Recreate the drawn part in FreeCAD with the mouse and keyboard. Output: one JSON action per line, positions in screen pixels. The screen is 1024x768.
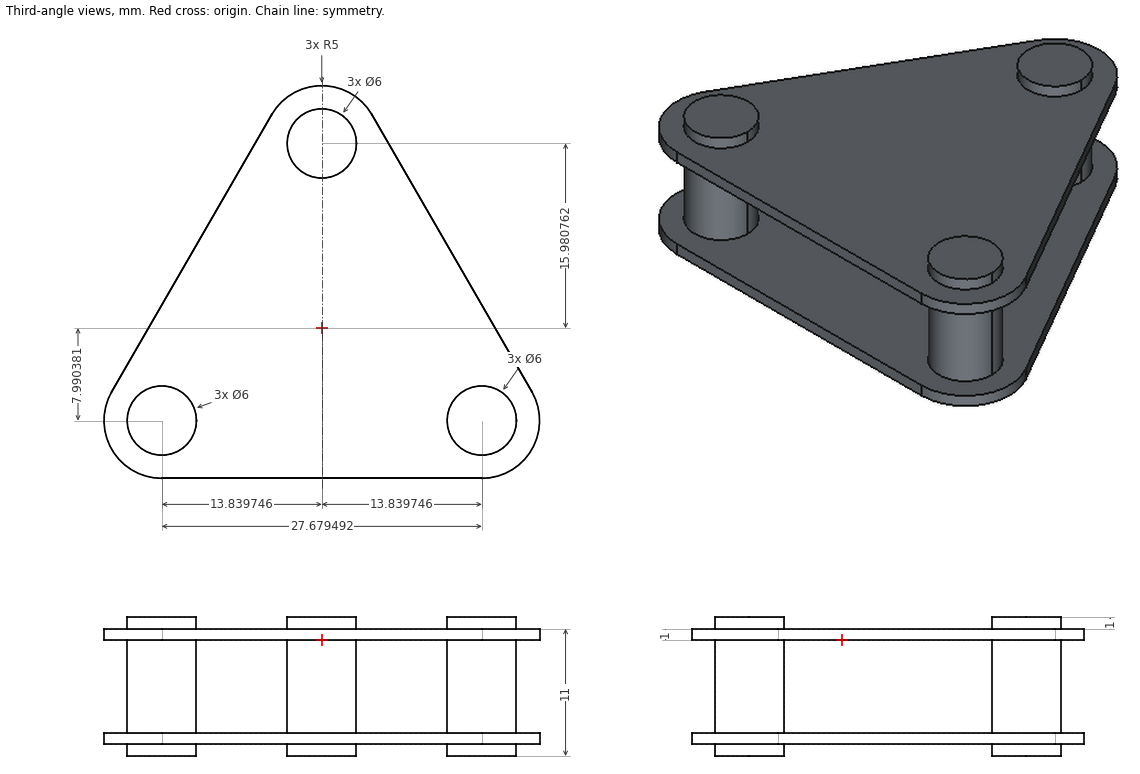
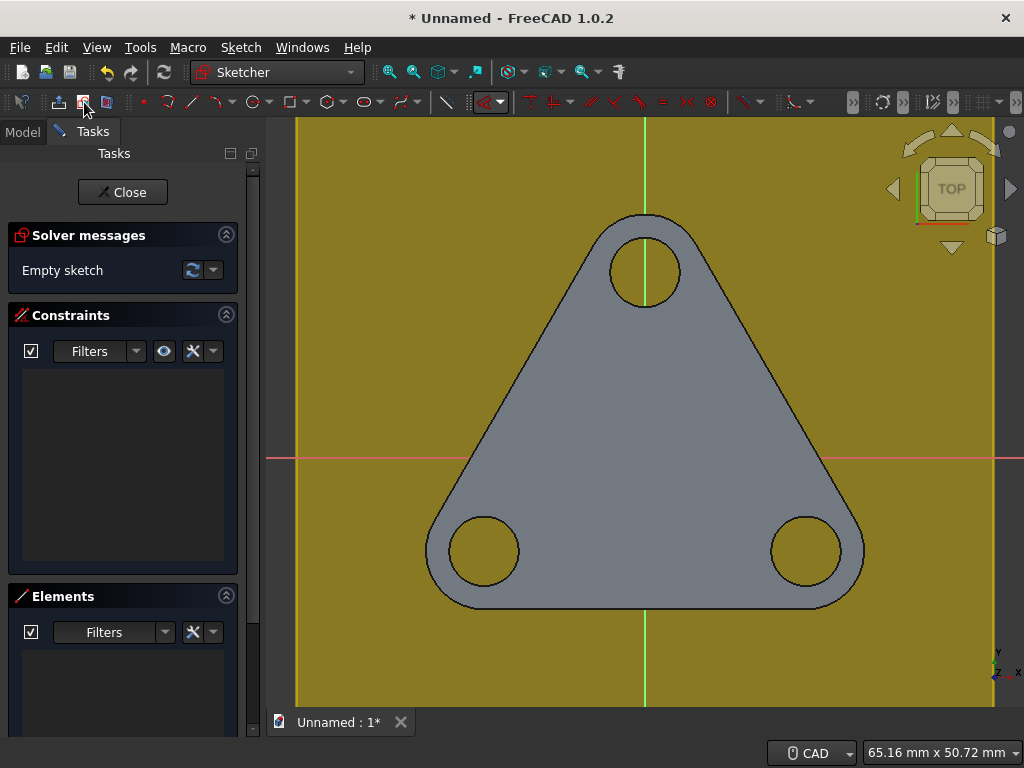
{"action": "left_click", "coordinate": [108, 102]}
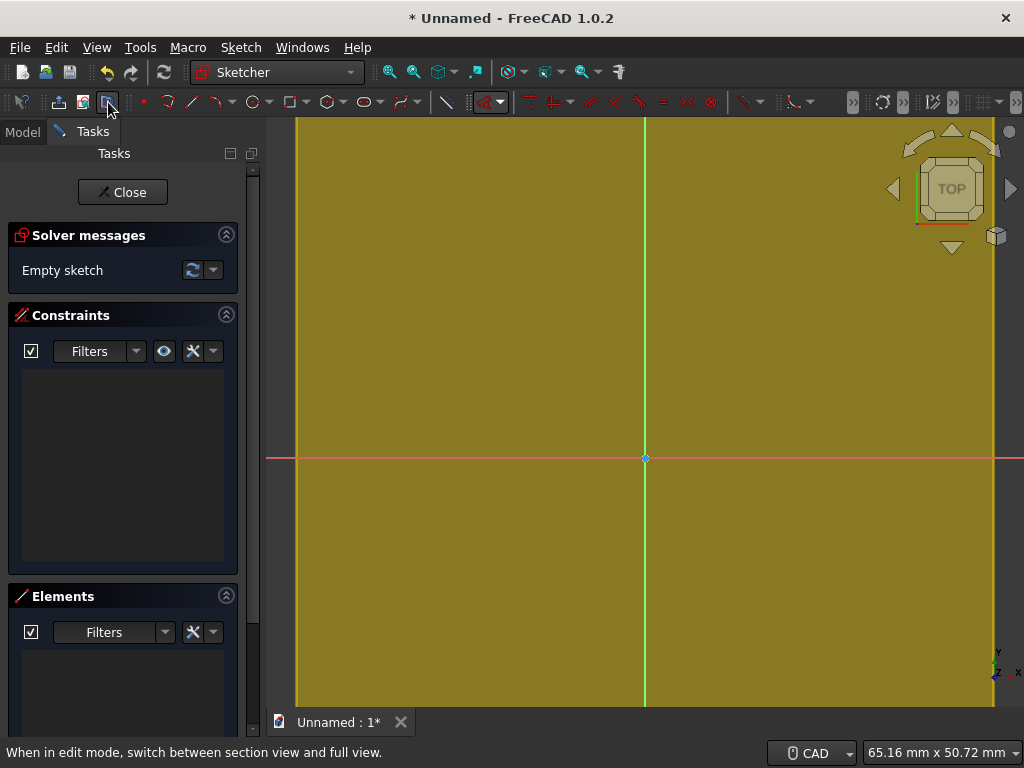
{"action": "scroll", "coordinate": [294, 413], "scroll_direction": "down", "scroll_amount": 1}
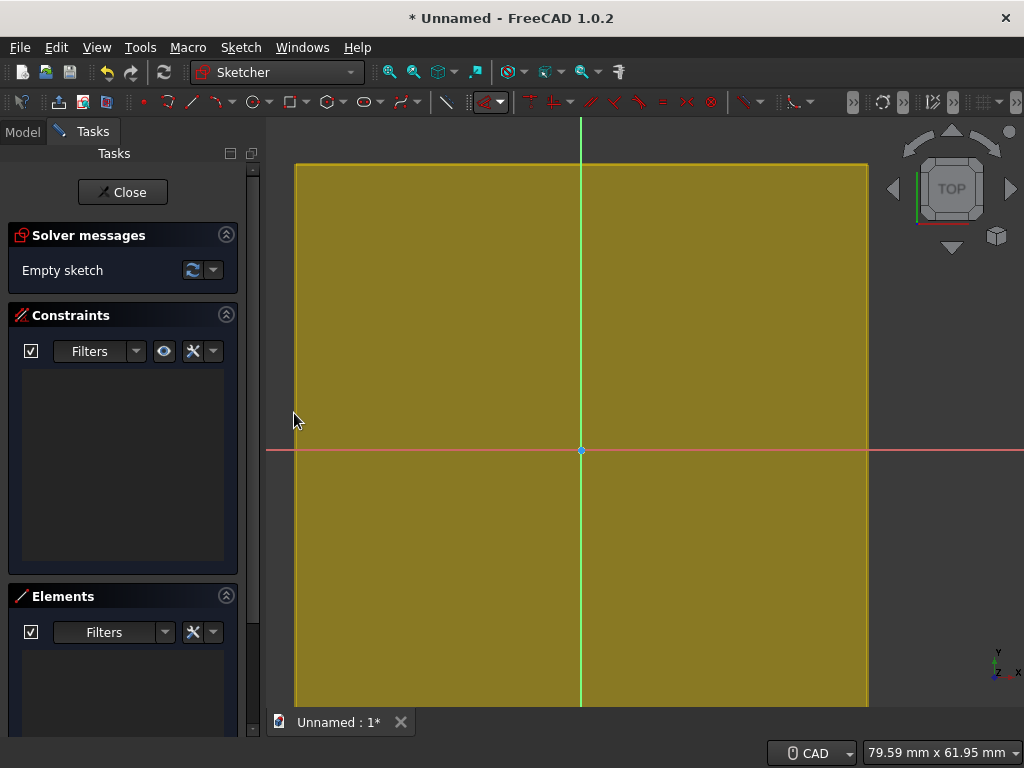
{"action": "left_click", "coordinate": [254, 102]}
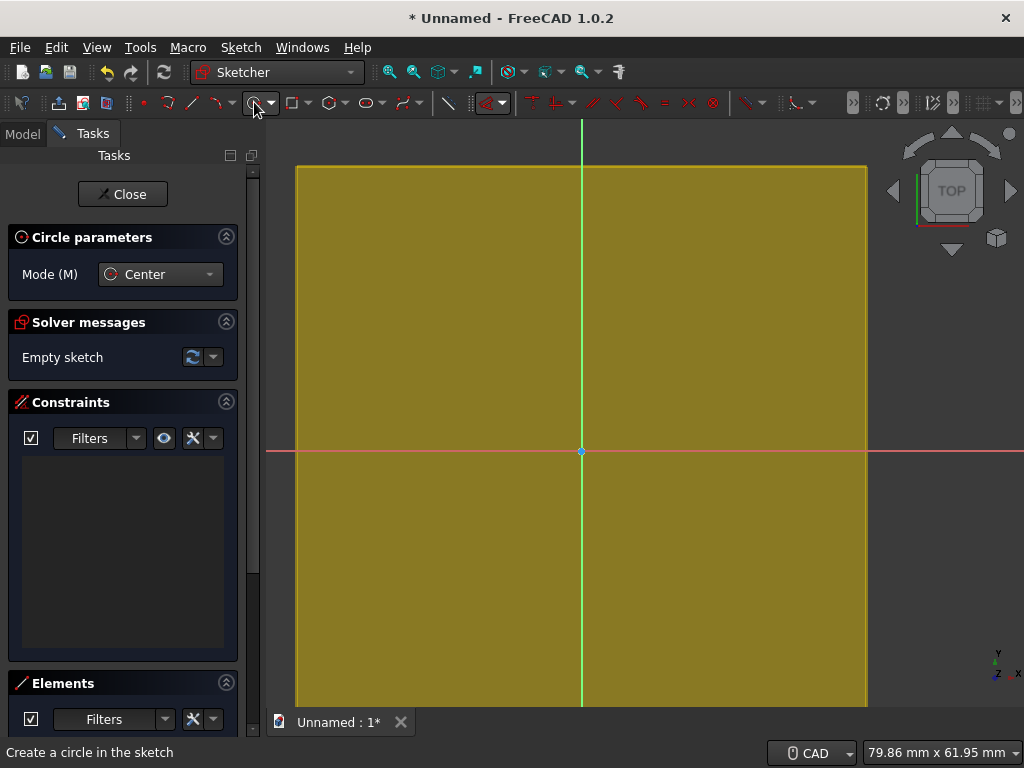
{"action": "left_click", "coordinate": [713, 527]}
{"action": "mouse_move", "coordinate": [733, 507]}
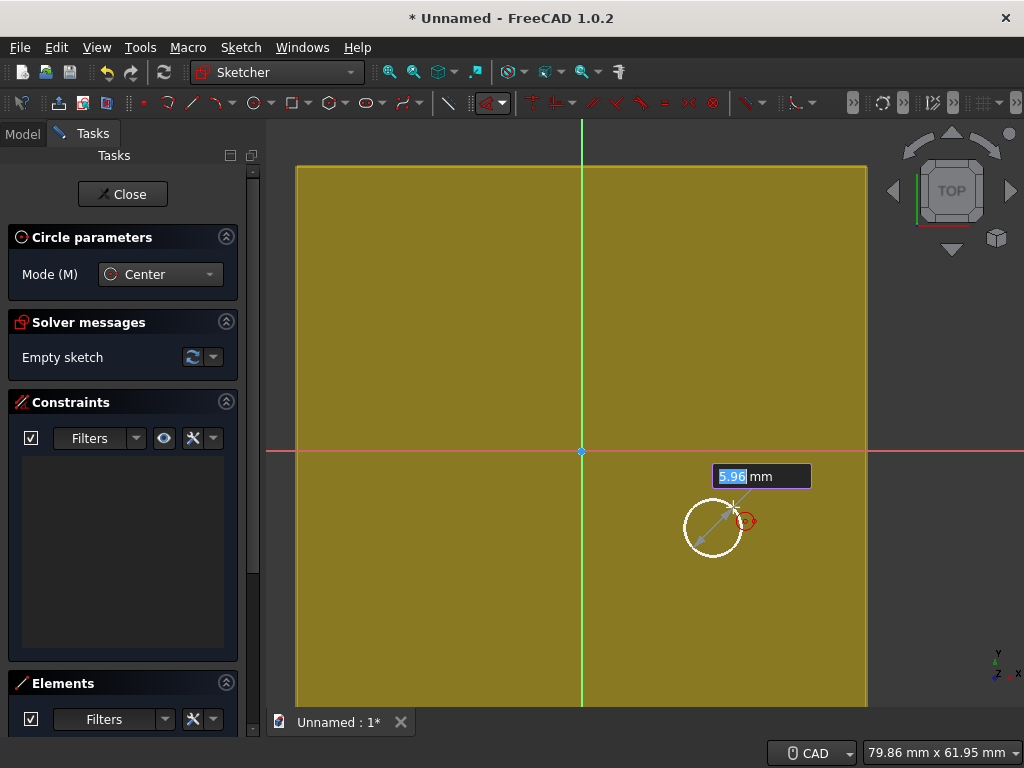
{"action": "type", "text": "6"}
{"action": "key", "text": "Return"}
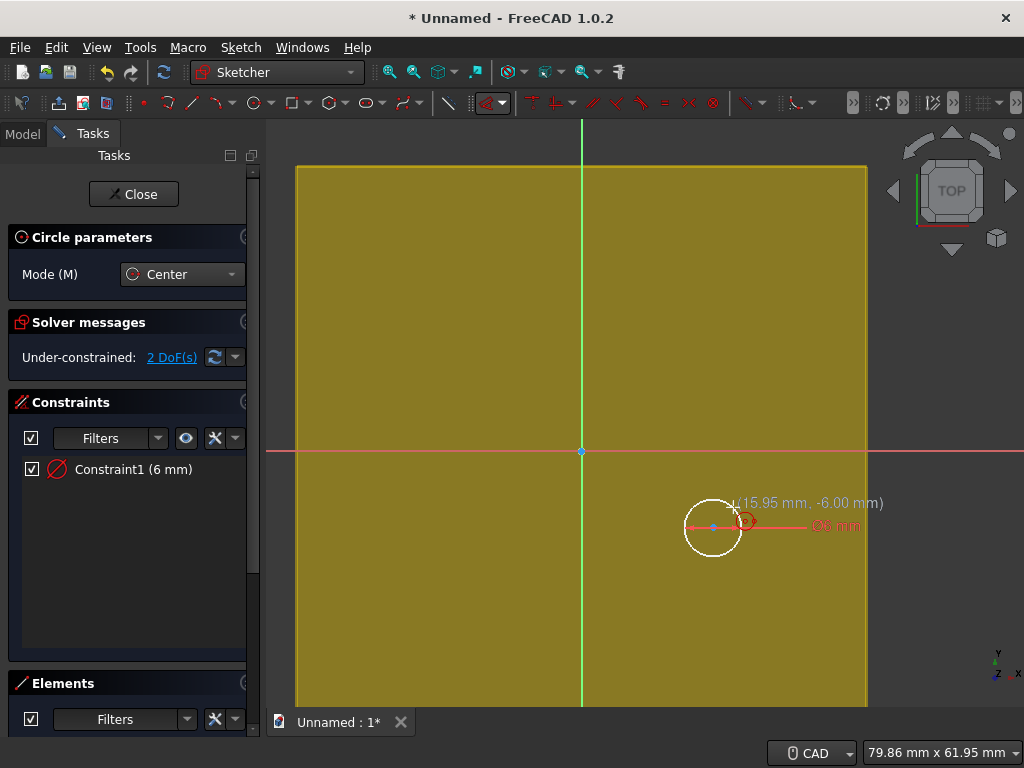
{"action": "left_click", "coordinate": [450, 527]}
{"action": "mouse_move", "coordinate": [470, 507]}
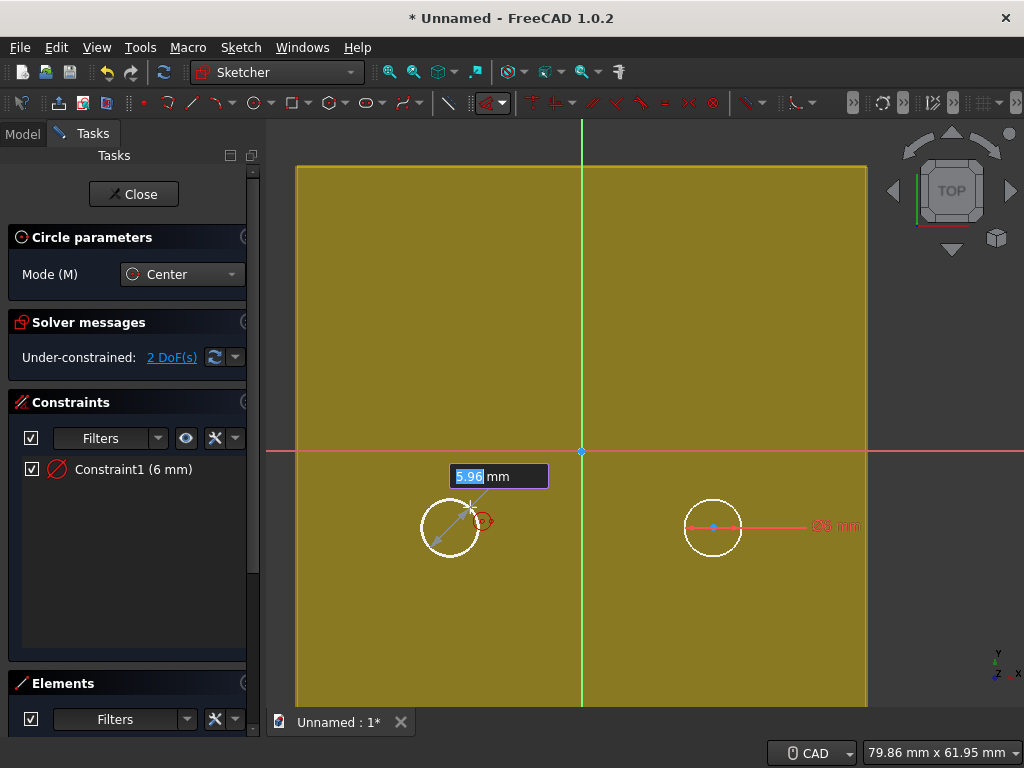
{"action": "type", "text": "6"}
{"action": "key", "text": "Return"}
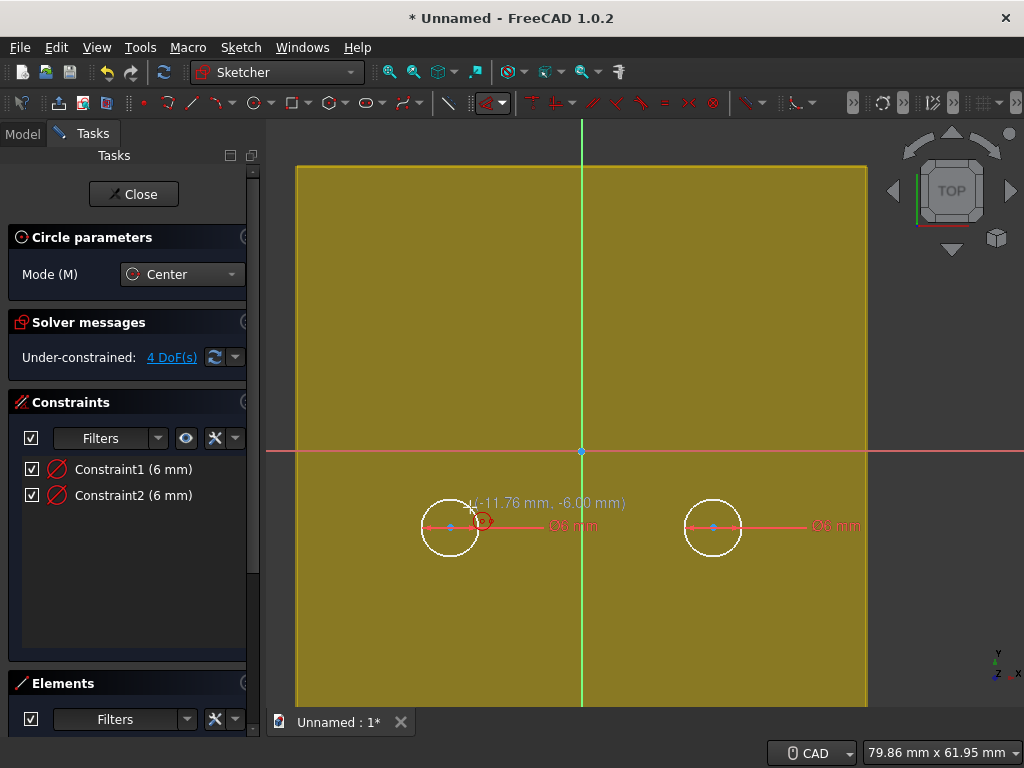
{"action": "left_click", "coordinate": [582, 299]}
{"action": "mouse_move", "coordinate": [602, 279]}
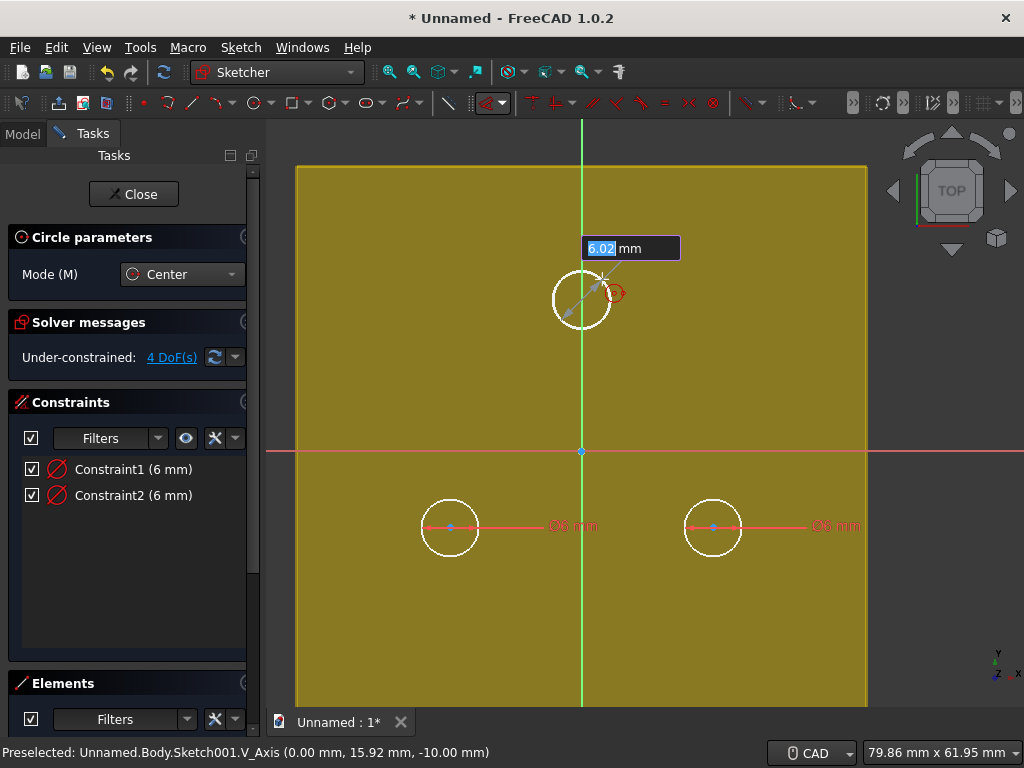
{"action": "type", "text": "6"}
{"action": "key", "text": "Return"}
{"action": "key", "text": "Escape"}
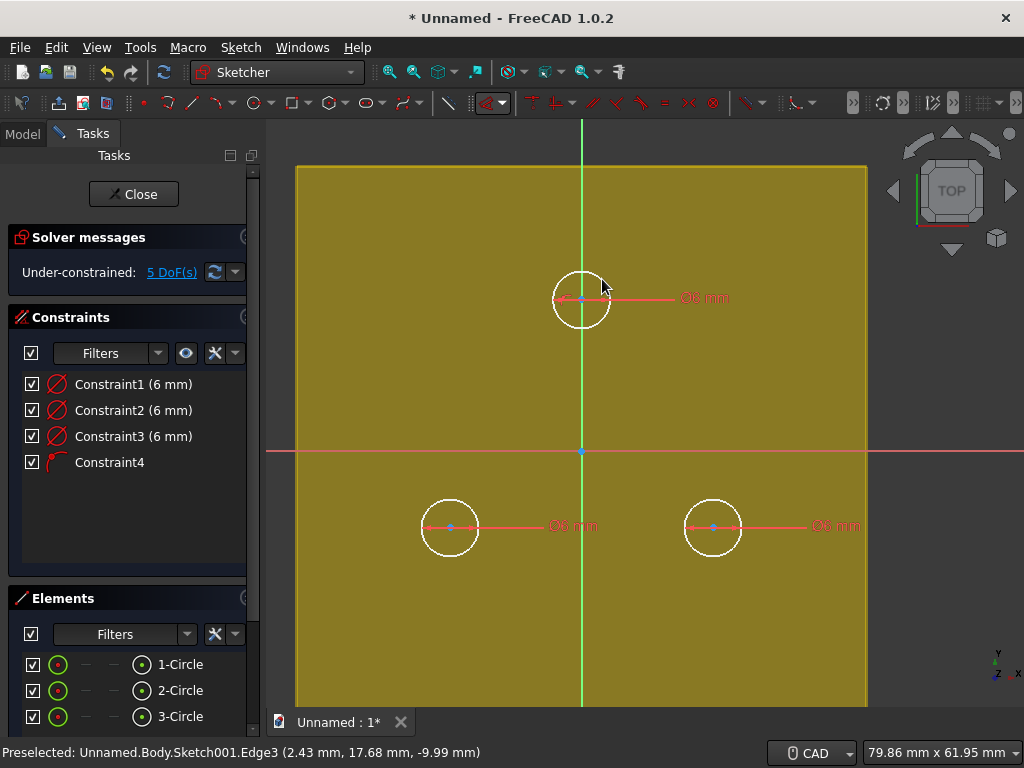
{"action": "left_click", "coordinate": [713, 528]}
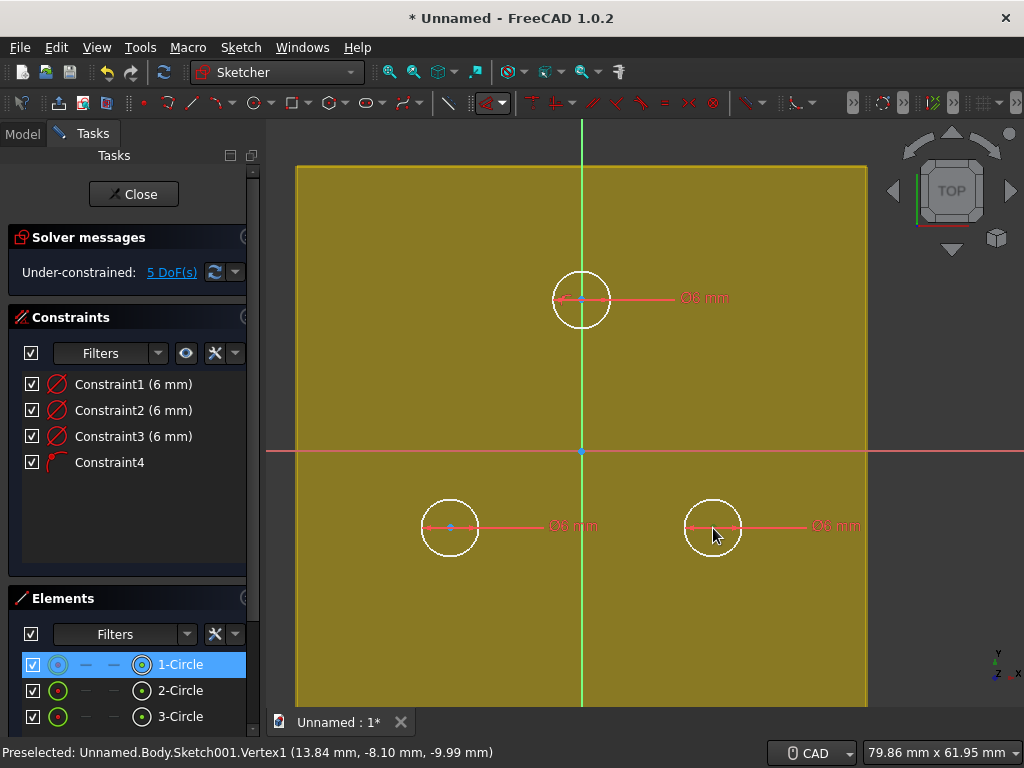
{"action": "left_click", "coordinate": [450, 528]}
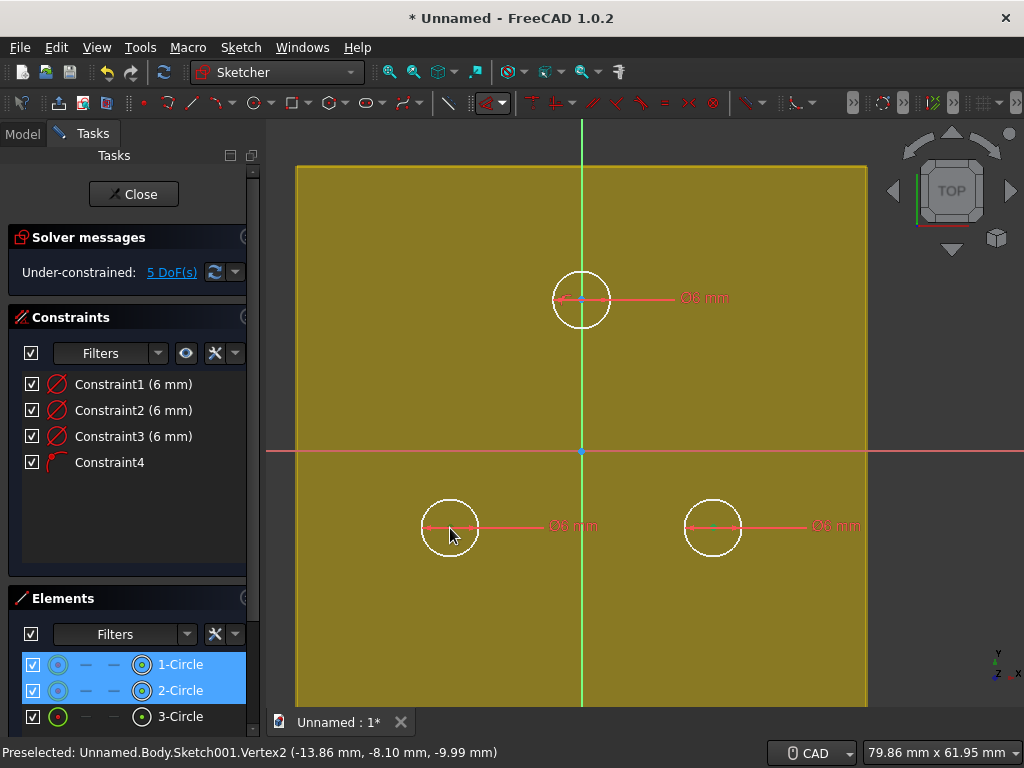
{"action": "left_click", "coordinate": [582, 641]}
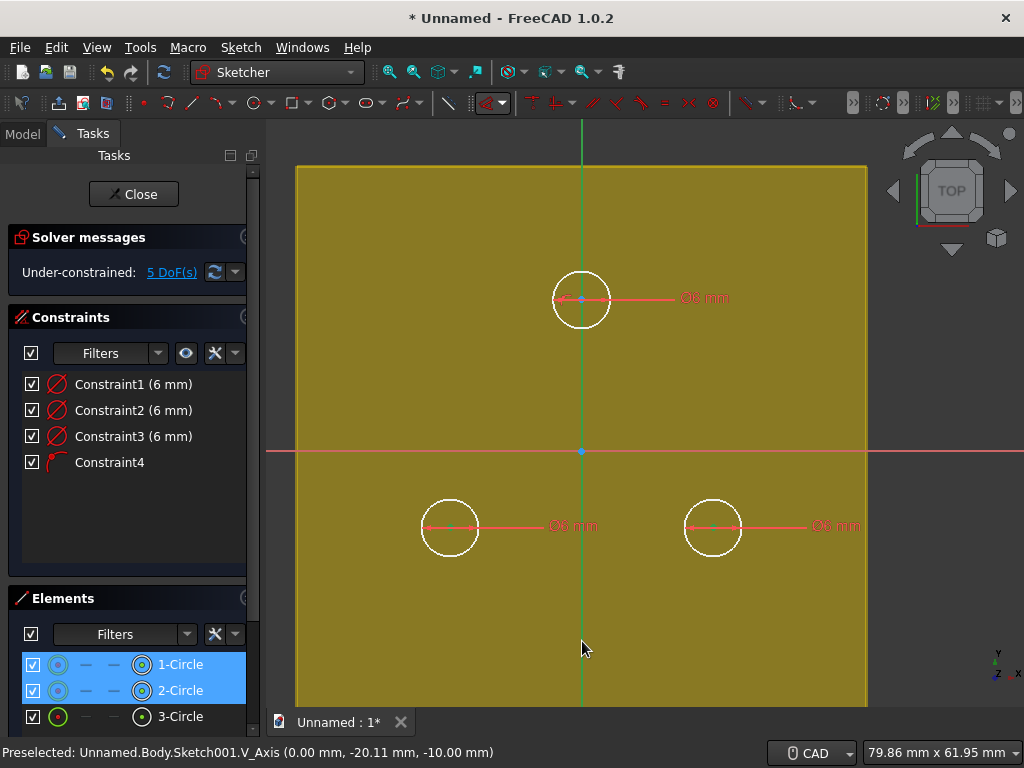
{"action": "left_click", "coordinate": [690, 104]}